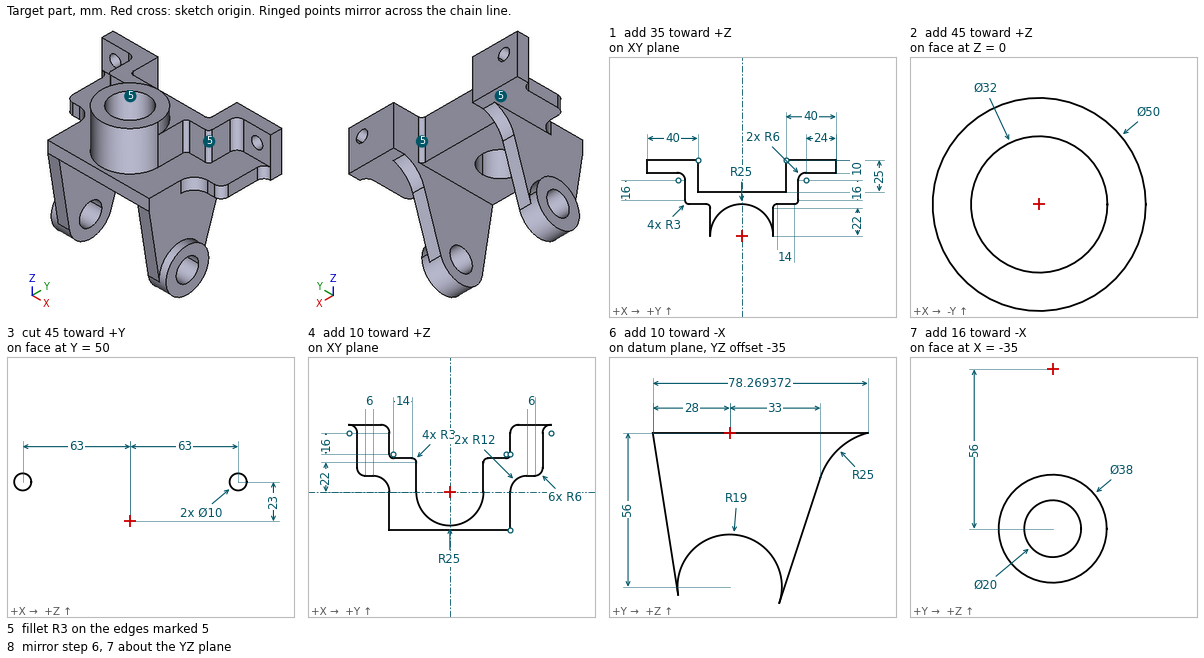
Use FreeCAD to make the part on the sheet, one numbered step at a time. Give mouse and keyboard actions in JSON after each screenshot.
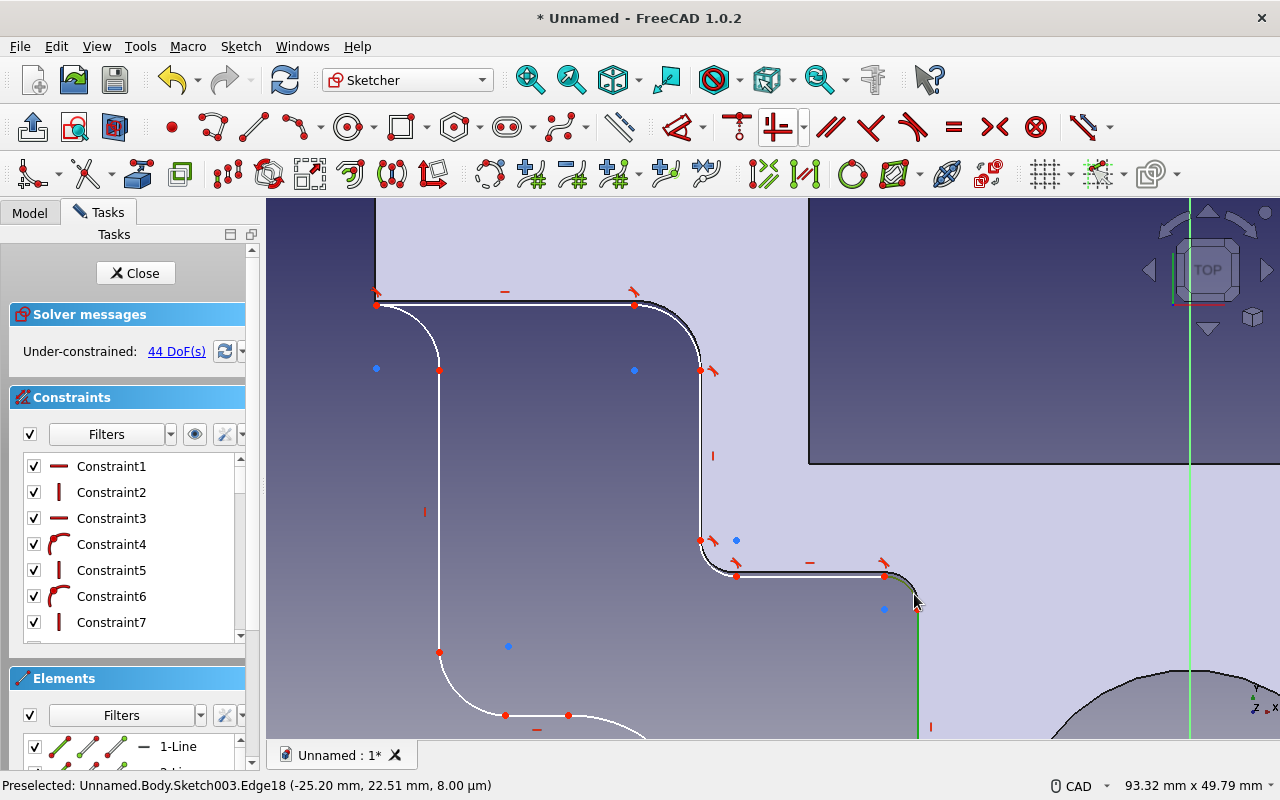
{"action": "left_click", "coordinate": [913, 128]}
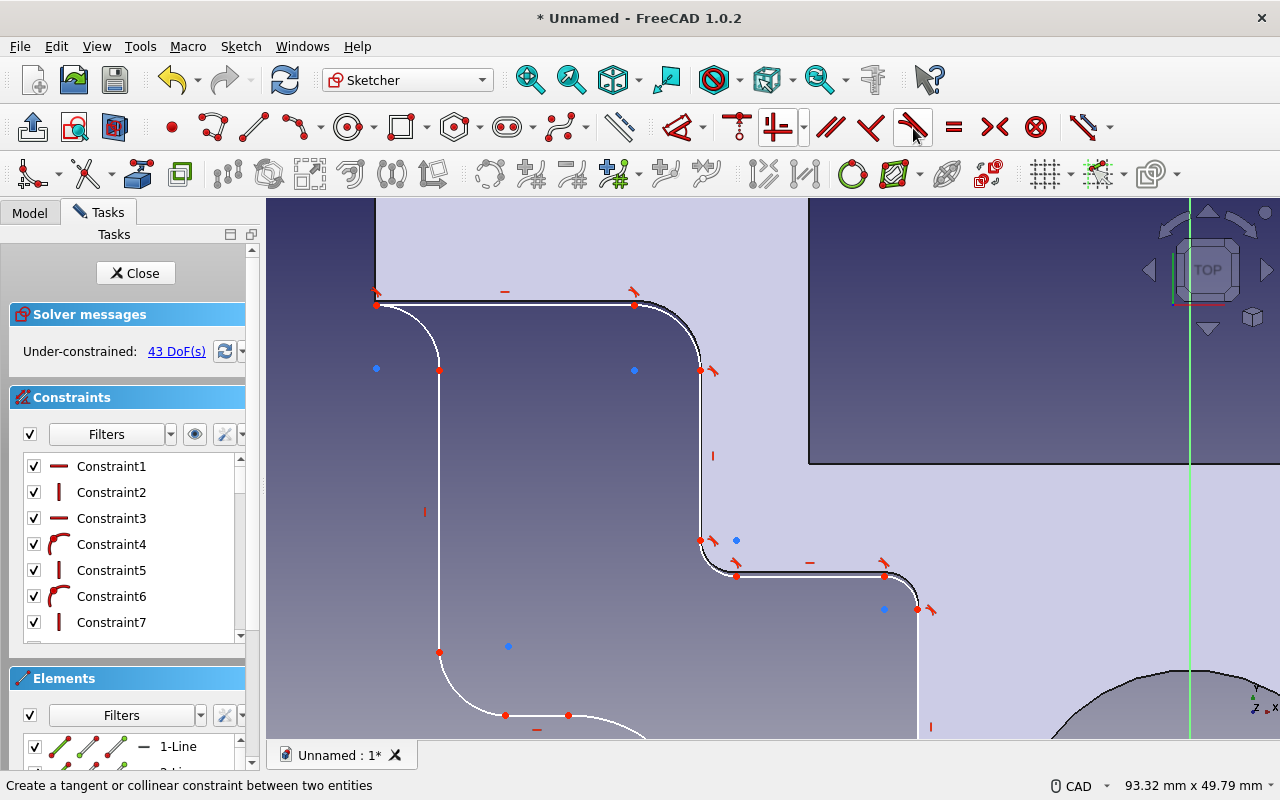
{"action": "left_click", "coordinate": [918, 680]}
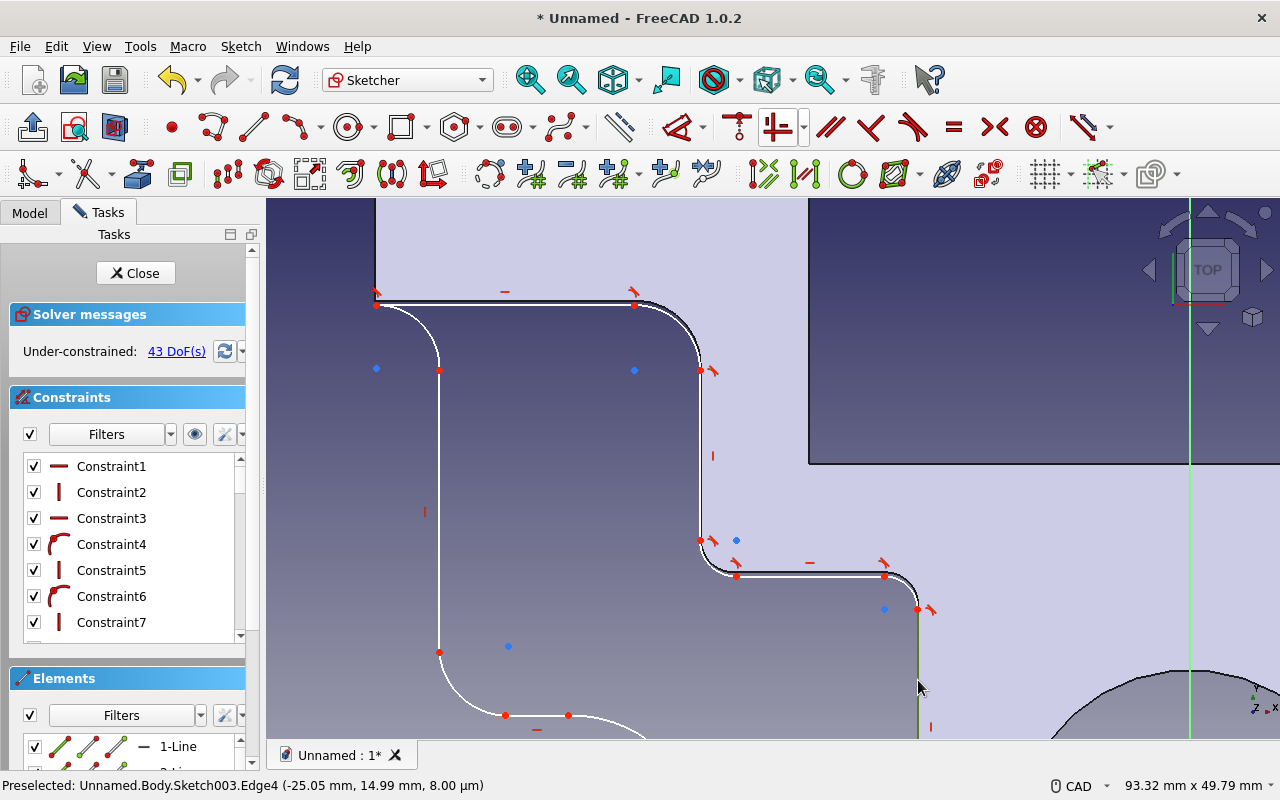
{"action": "scroll", "coordinate": [422, 320], "scroll_direction": "down", "scroll_amount": 5}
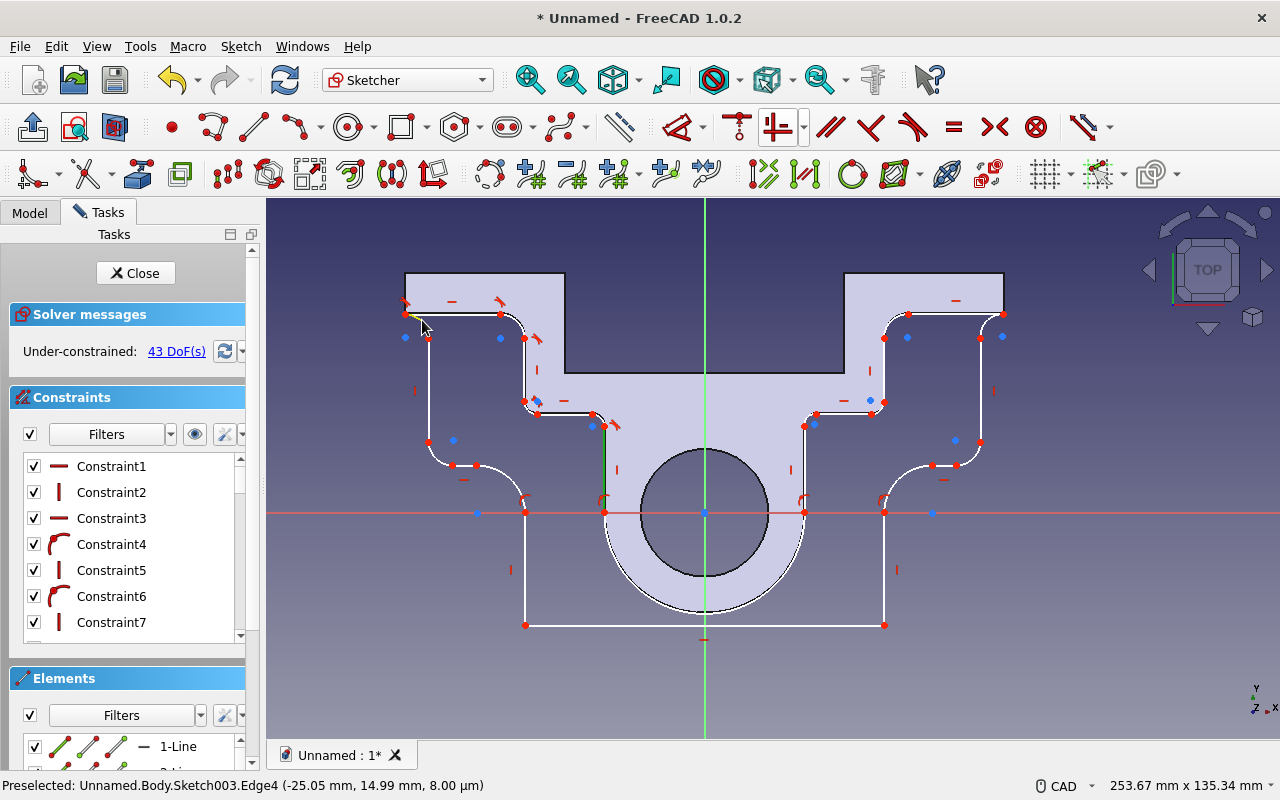
{"action": "left_click", "coordinate": [645, 595]}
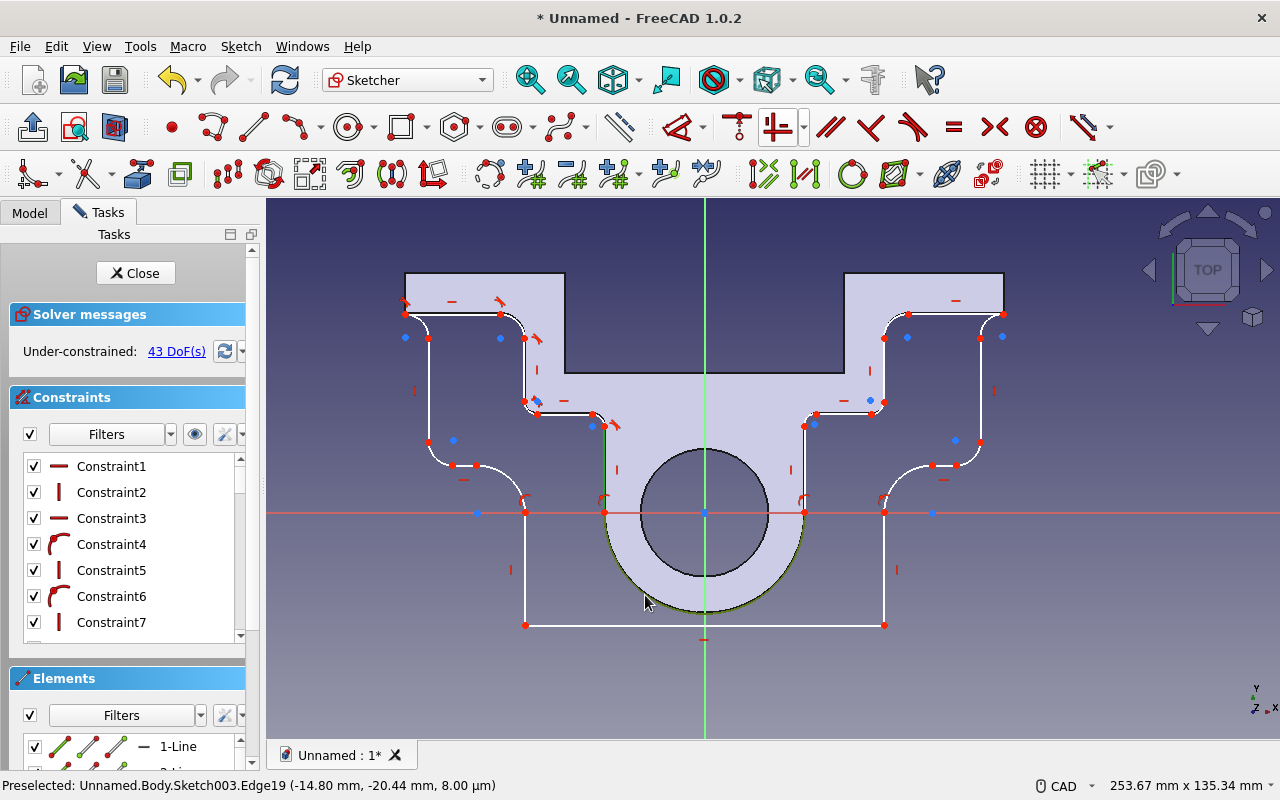
{"action": "left_click", "coordinate": [913, 128]}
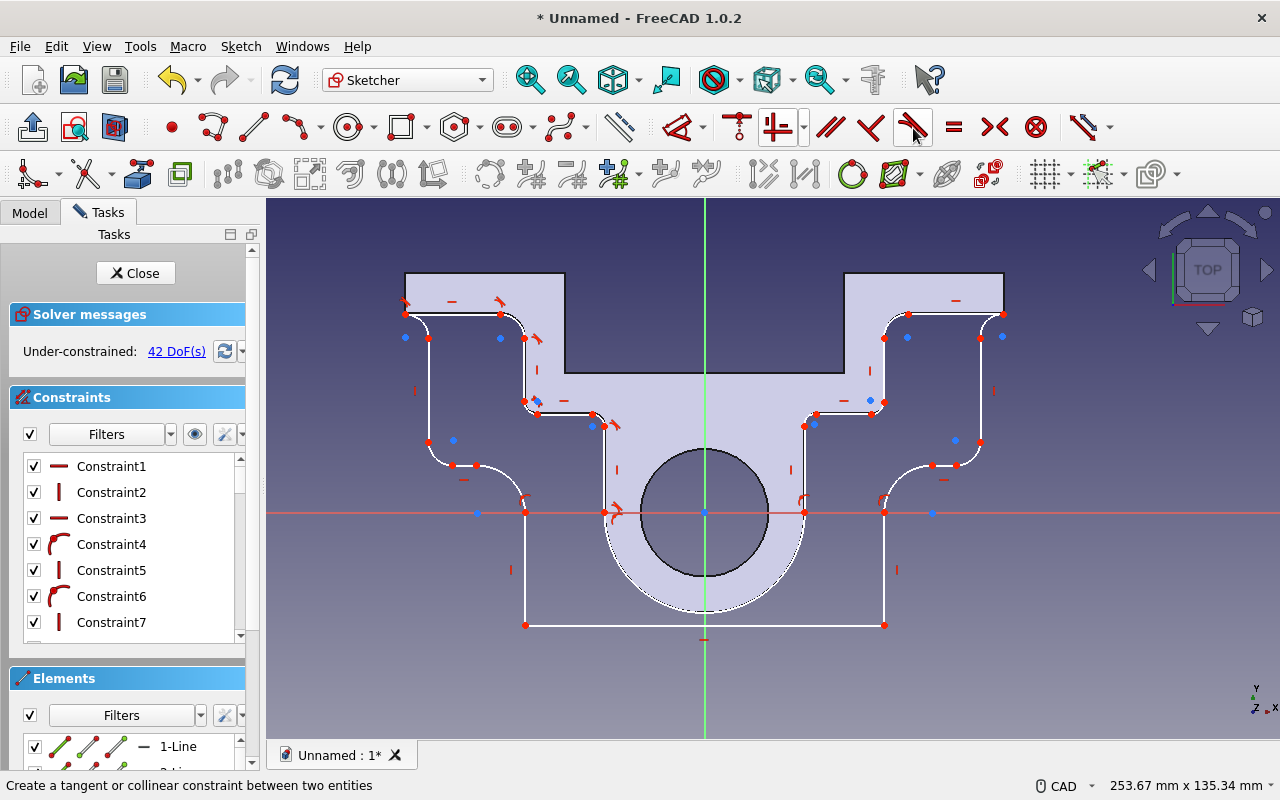
{"action": "left_click", "coordinate": [805, 487]}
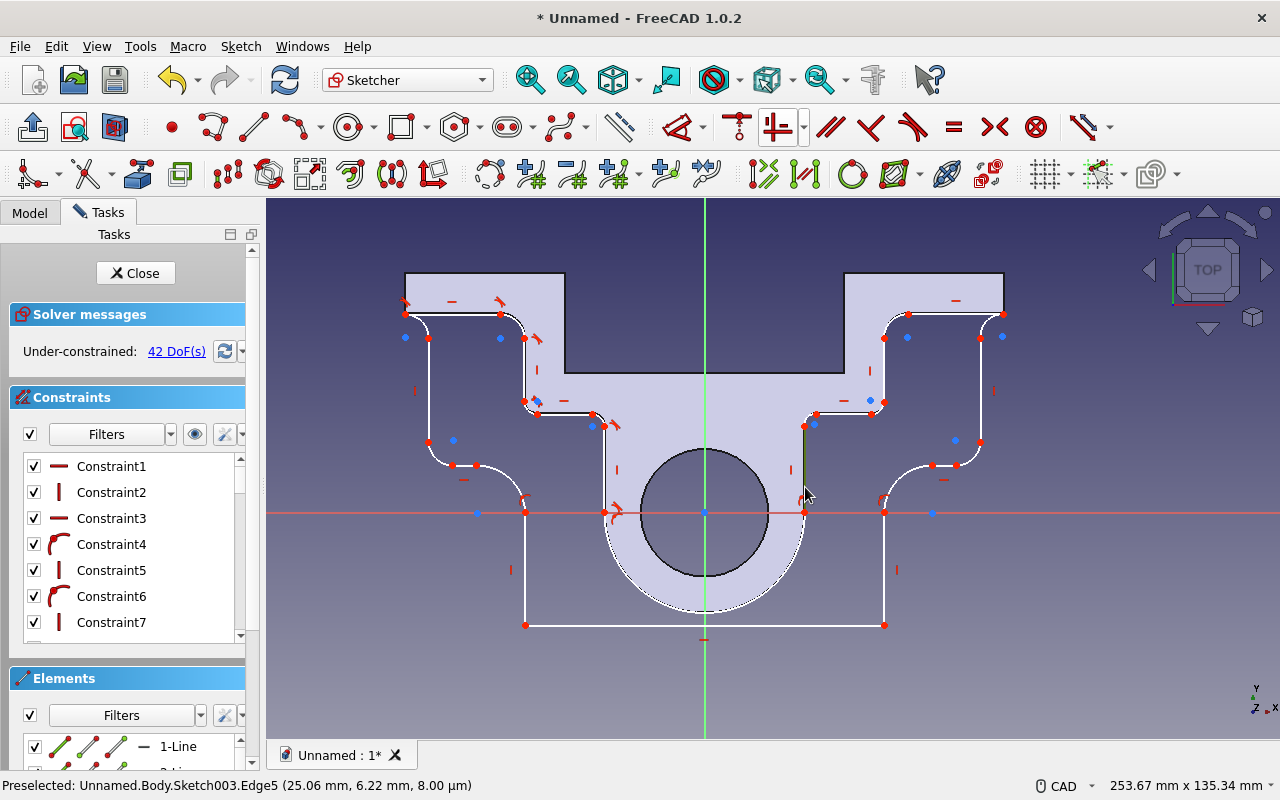
{"action": "scroll", "coordinate": [807, 417], "scroll_direction": "up", "scroll_amount": 2}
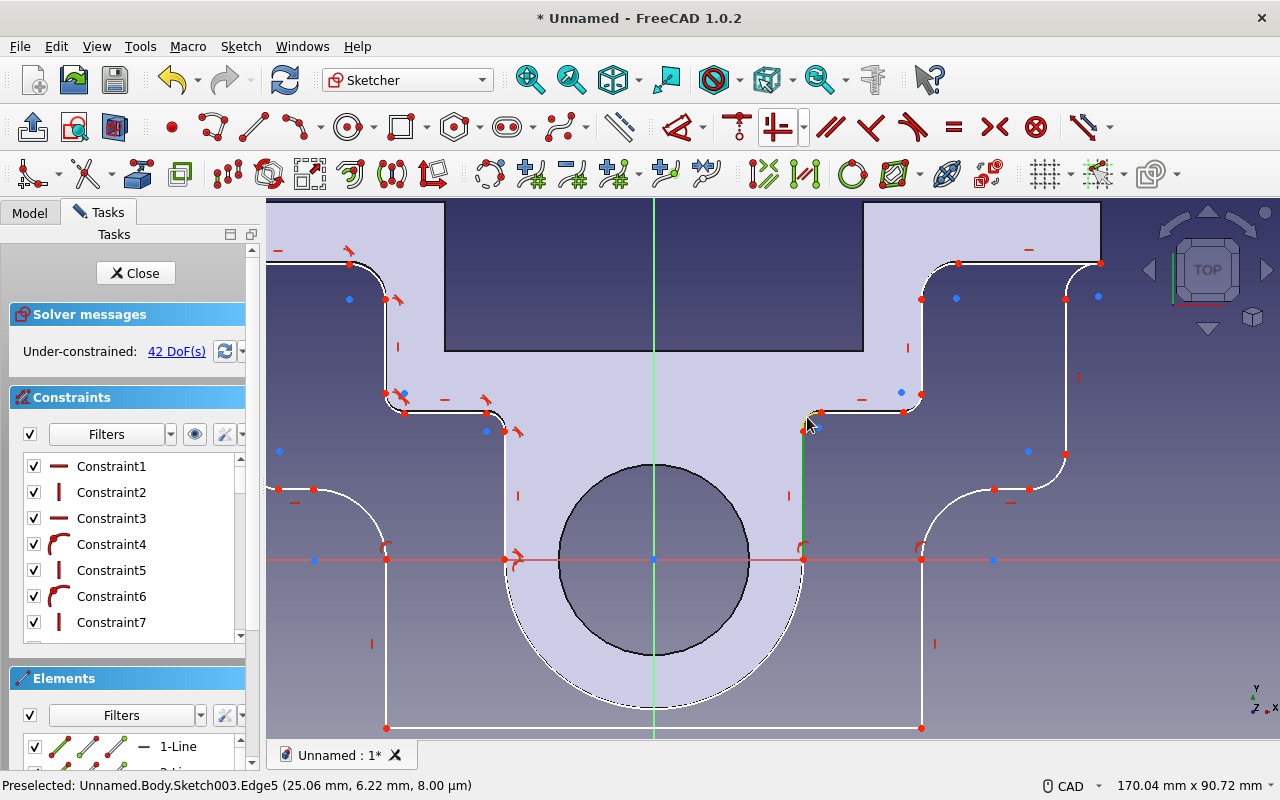
{"action": "left_click", "coordinate": [807, 417]}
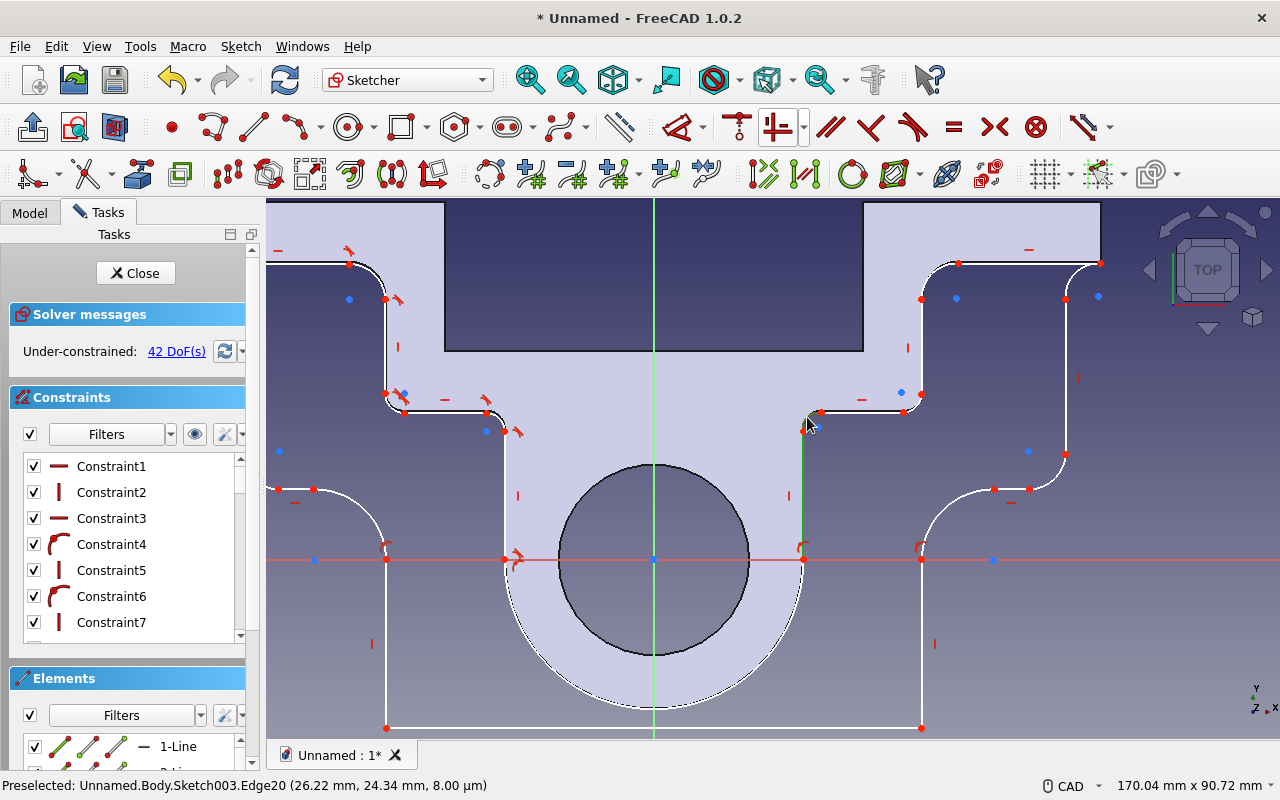
{"action": "left_click", "coordinate": [913, 128]}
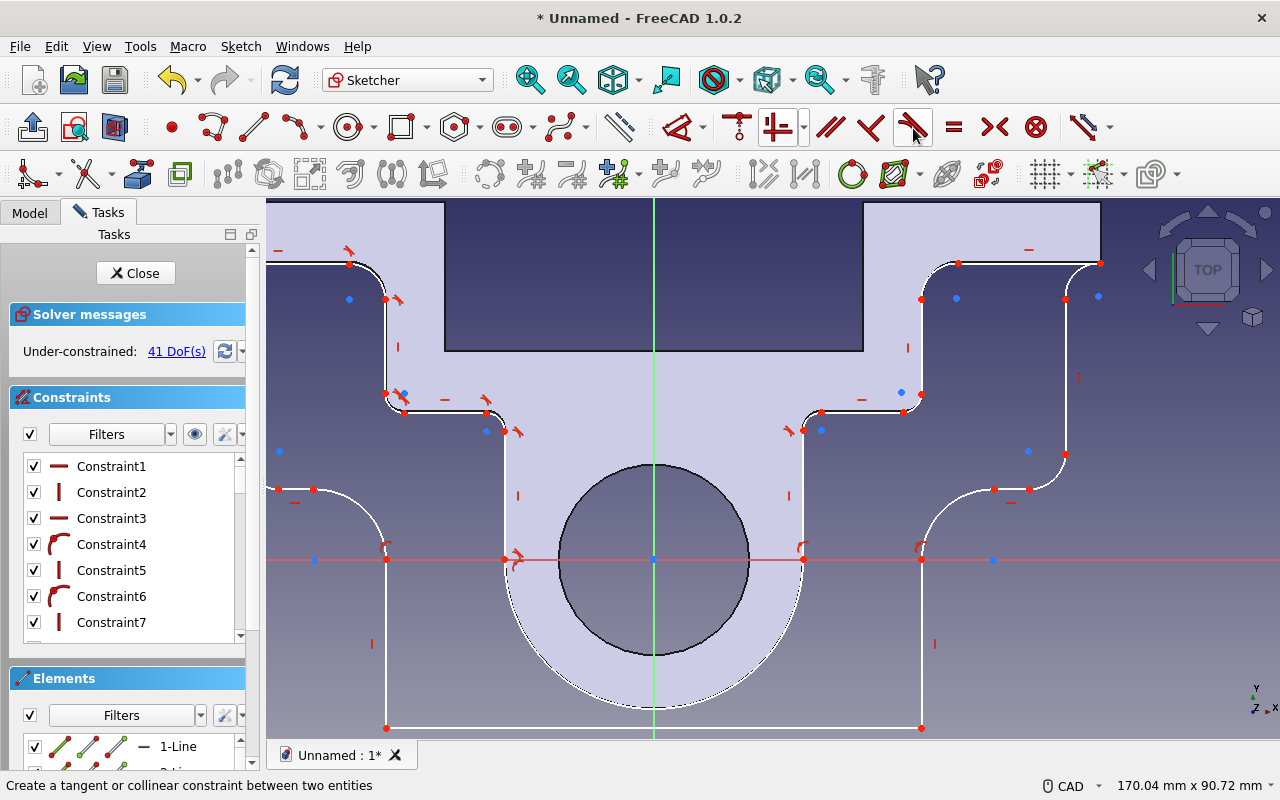
{"action": "left_click", "coordinate": [846, 413]}